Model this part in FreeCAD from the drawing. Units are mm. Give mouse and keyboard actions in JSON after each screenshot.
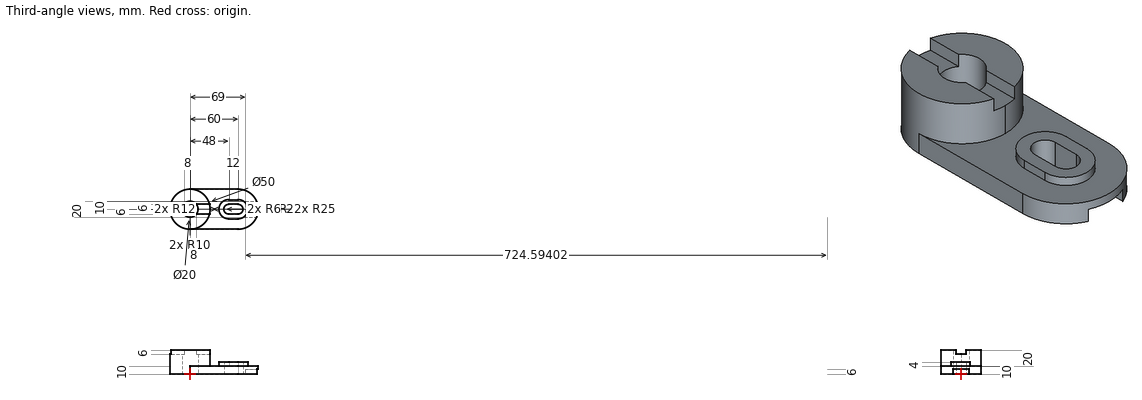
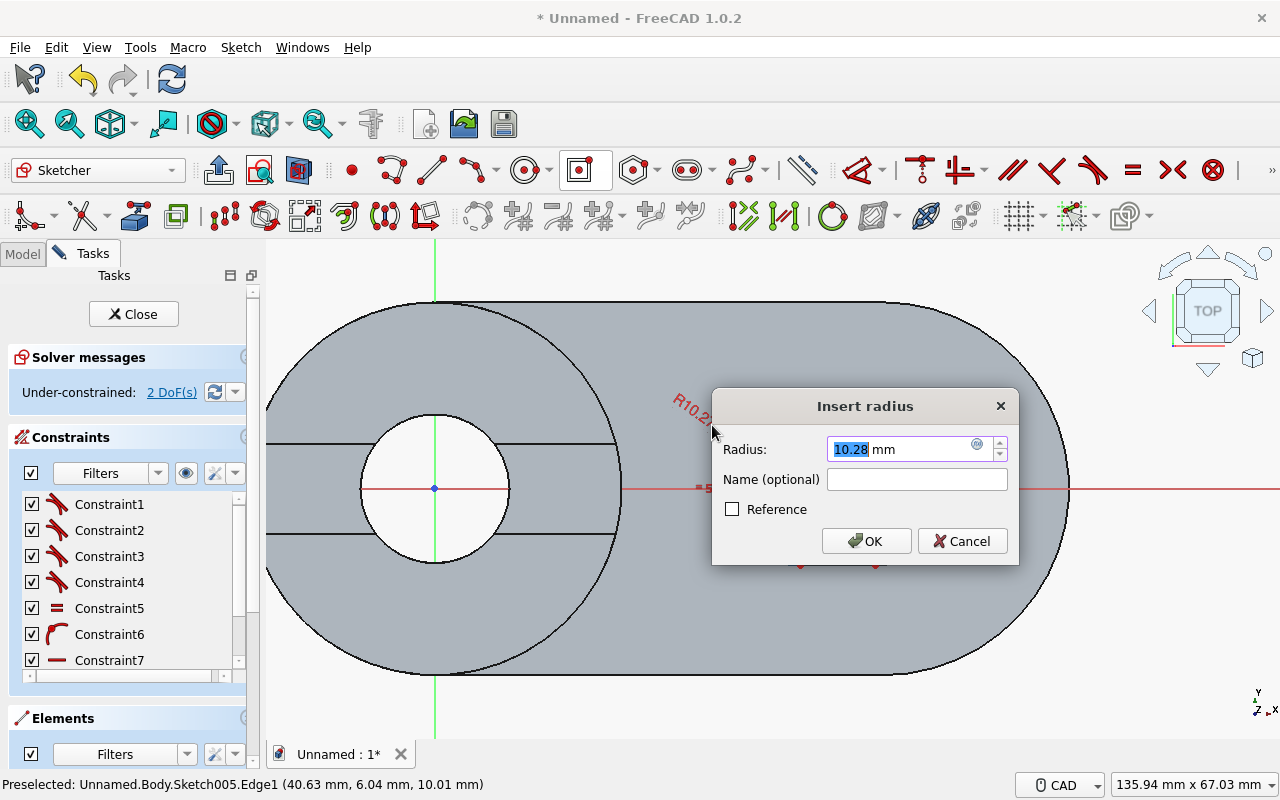
{"action": "type", "text": "12"}
{"action": "key", "text": "Return"}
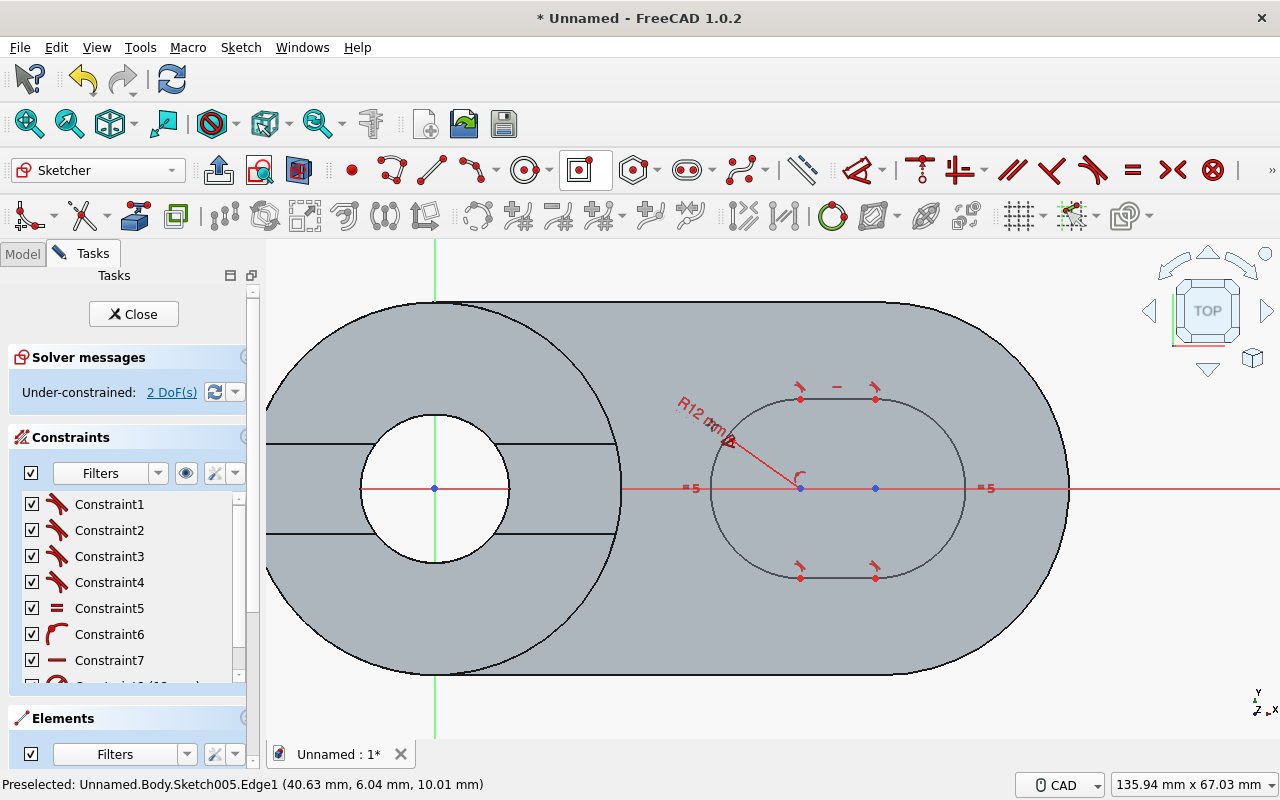
{"action": "left_click", "coordinate": [823, 399]}
{"action": "left_click", "coordinate": [838, 365]}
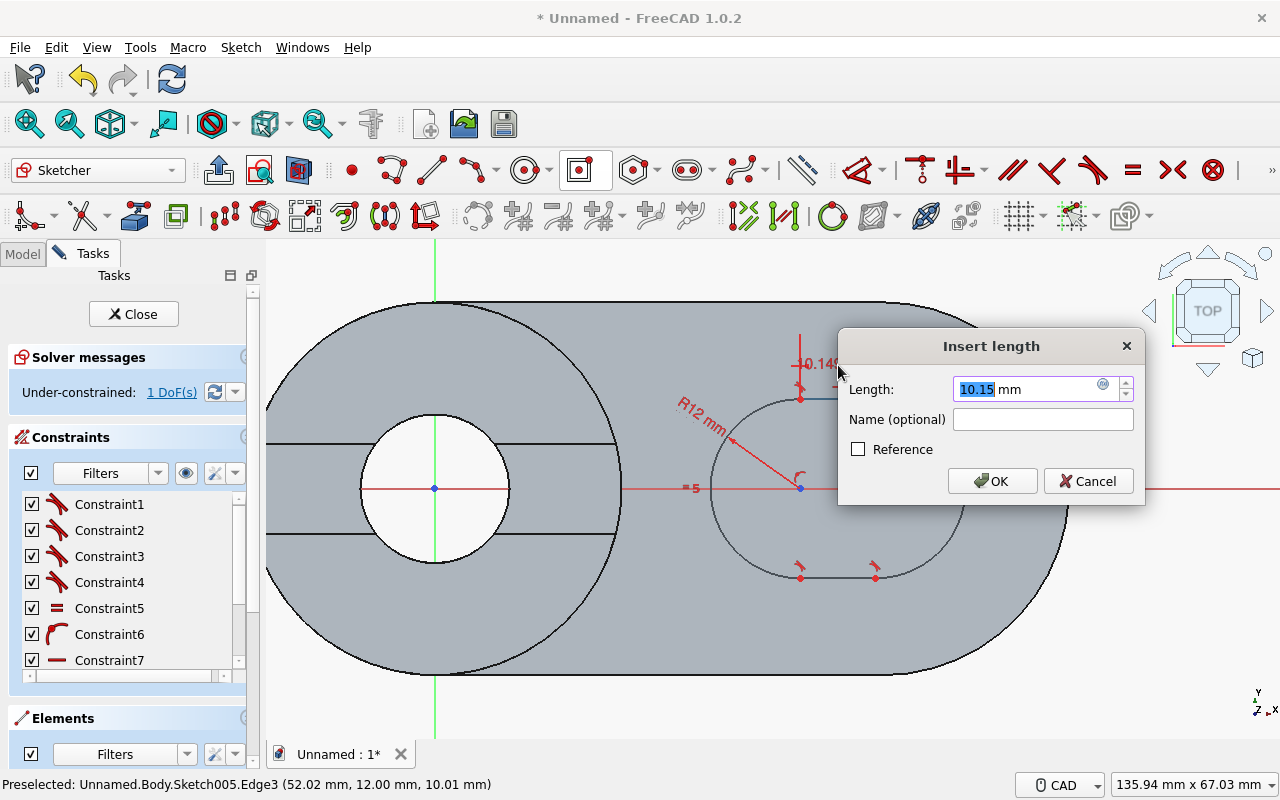
{"action": "type", "text": "12"}
{"action": "key", "text": "Return"}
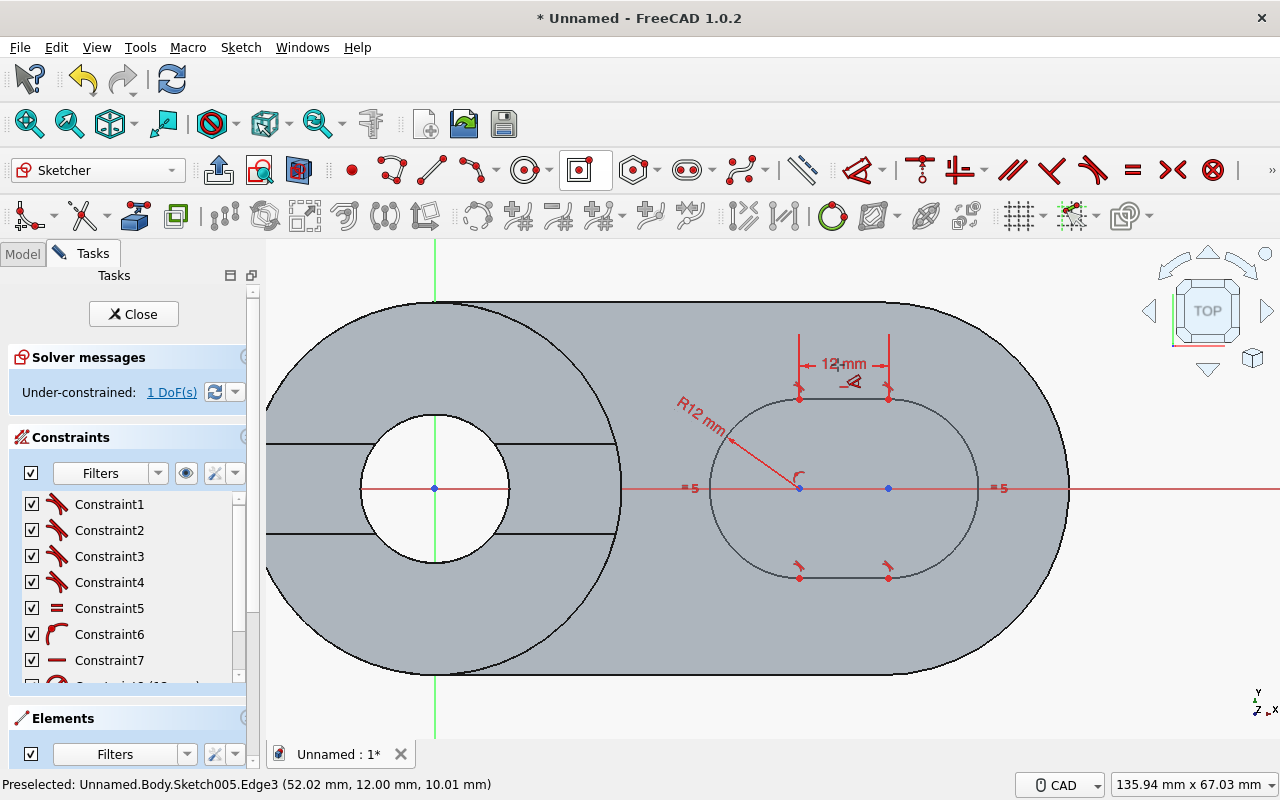
{"action": "left_click", "coordinate": [799, 399]}
{"action": "left_click", "coordinate": [617, 365]}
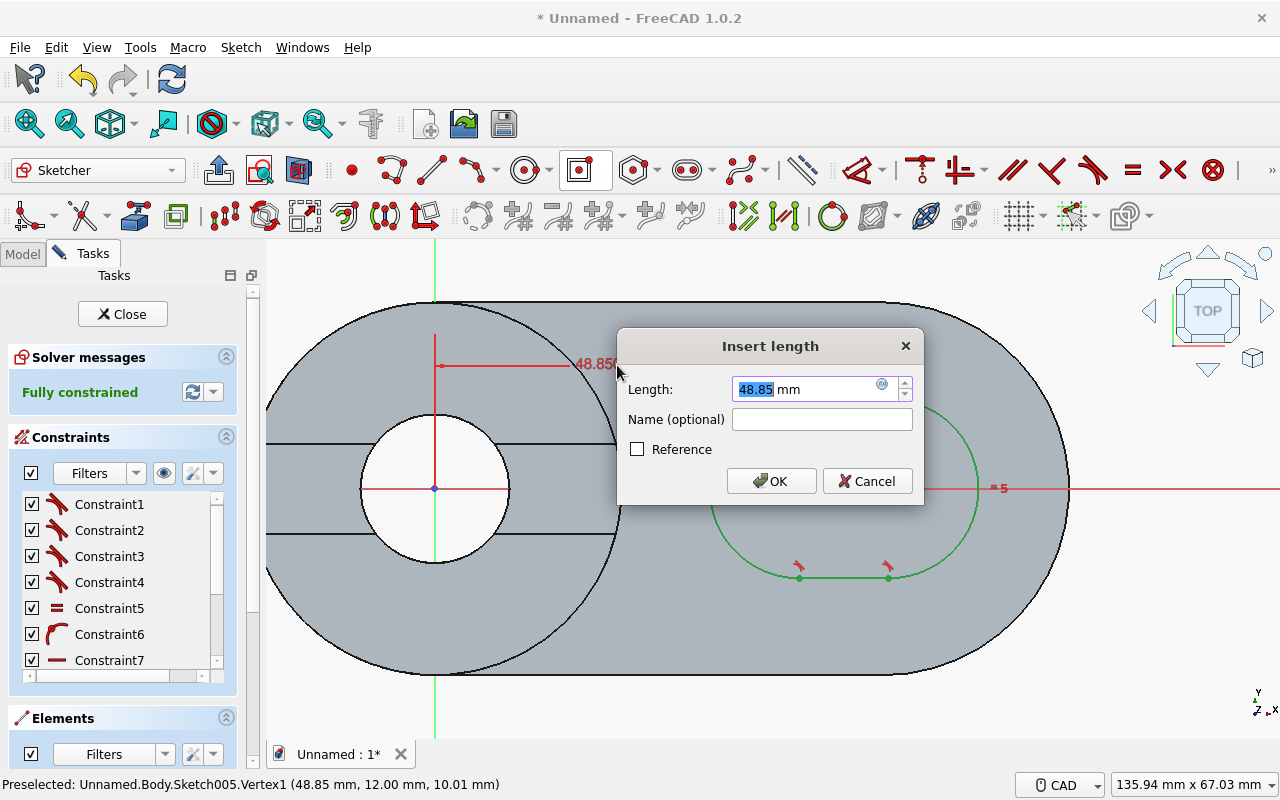
{"action": "type", "text": "48"}
{"action": "key", "text": "Return"}
{"action": "key", "text": "Escape"}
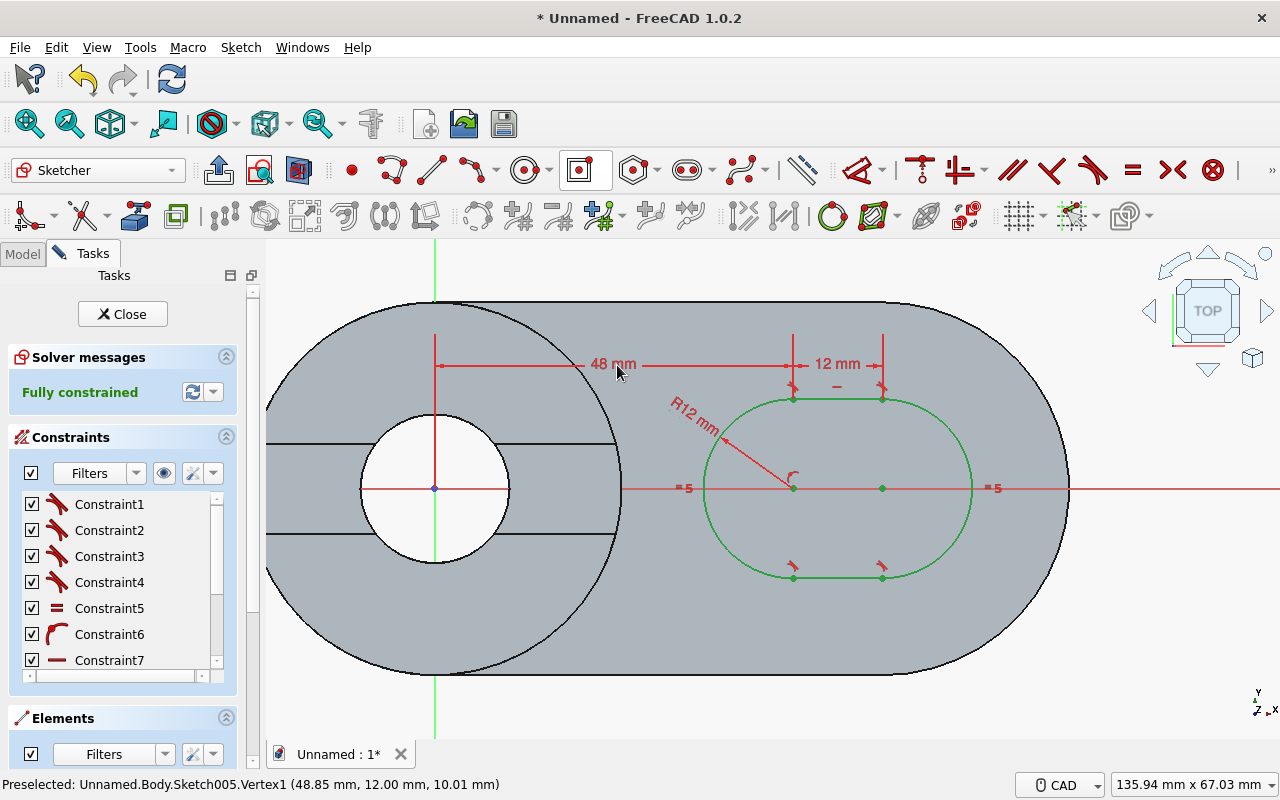
{"action": "left_click", "coordinate": [123, 314]}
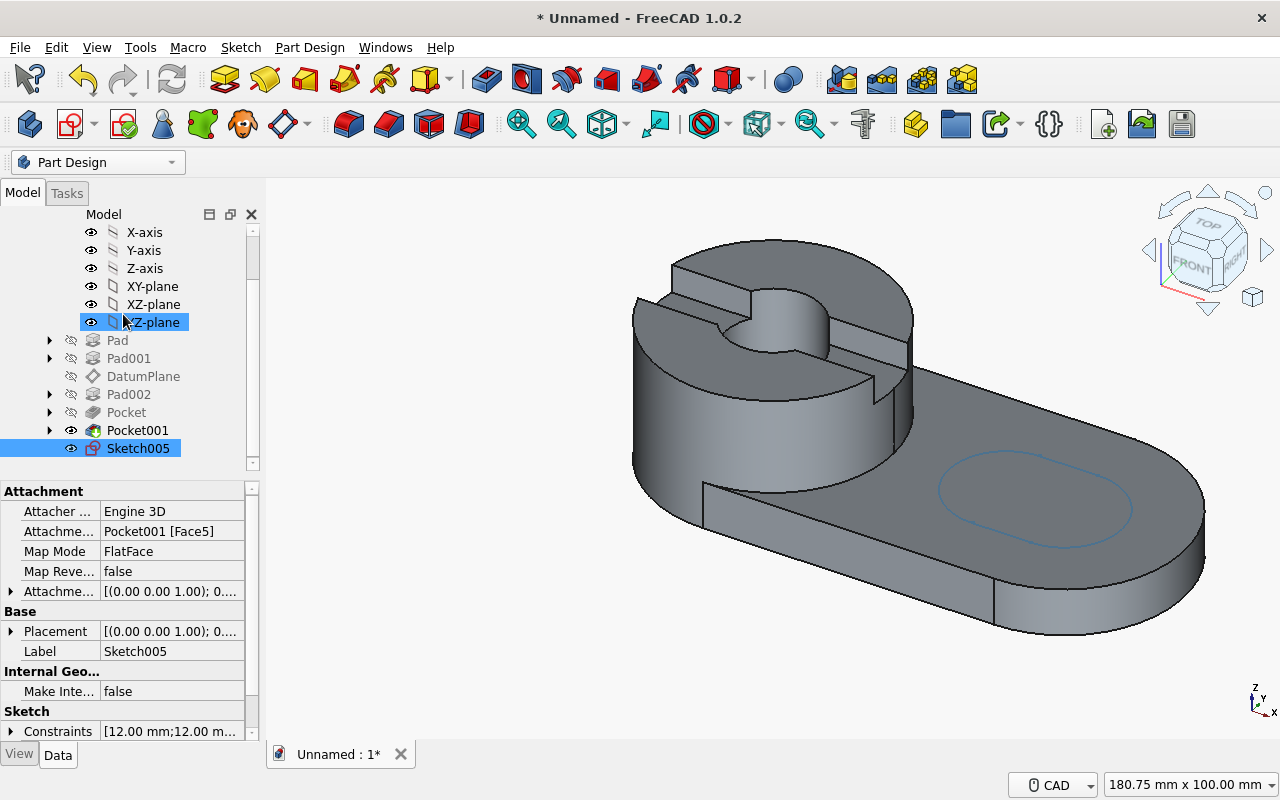
{"action": "left_click", "coordinate": [226, 80]}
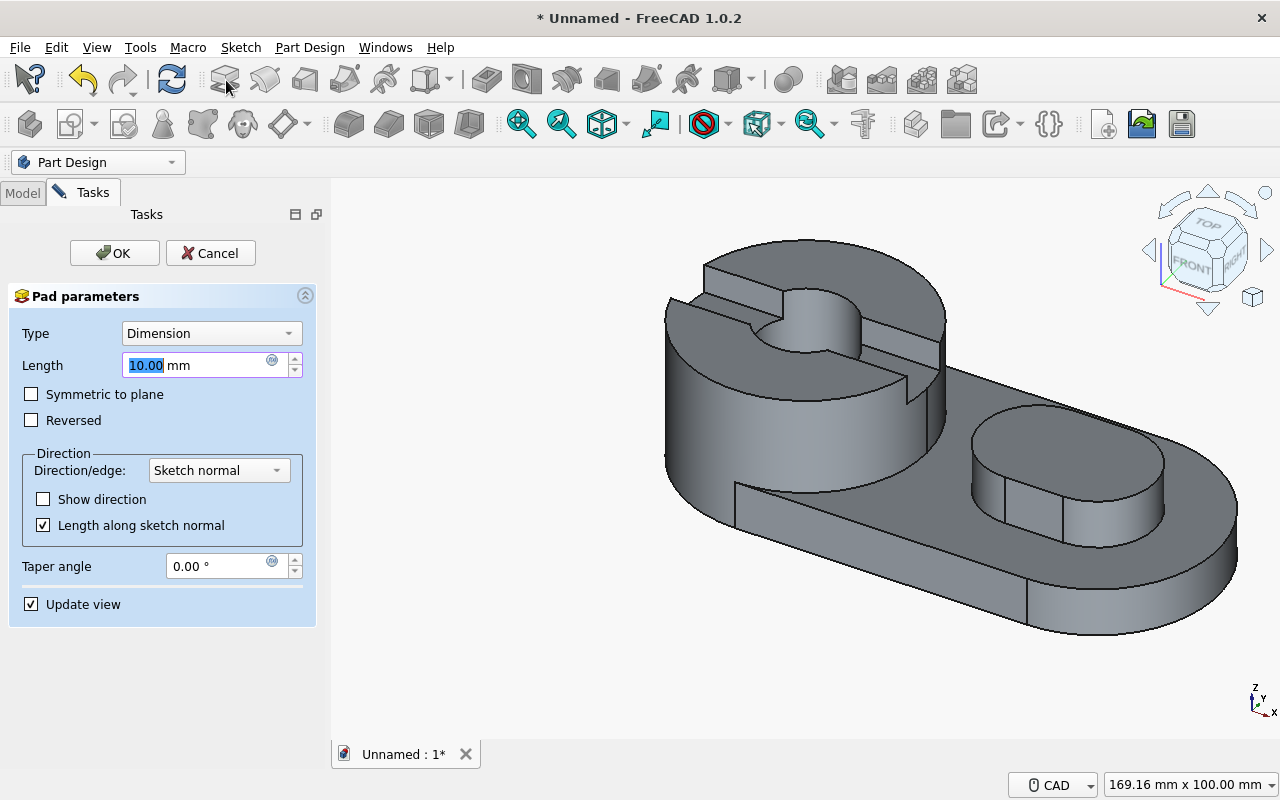
{"action": "type", "text": "4"}
{"action": "key", "text": "Tab"}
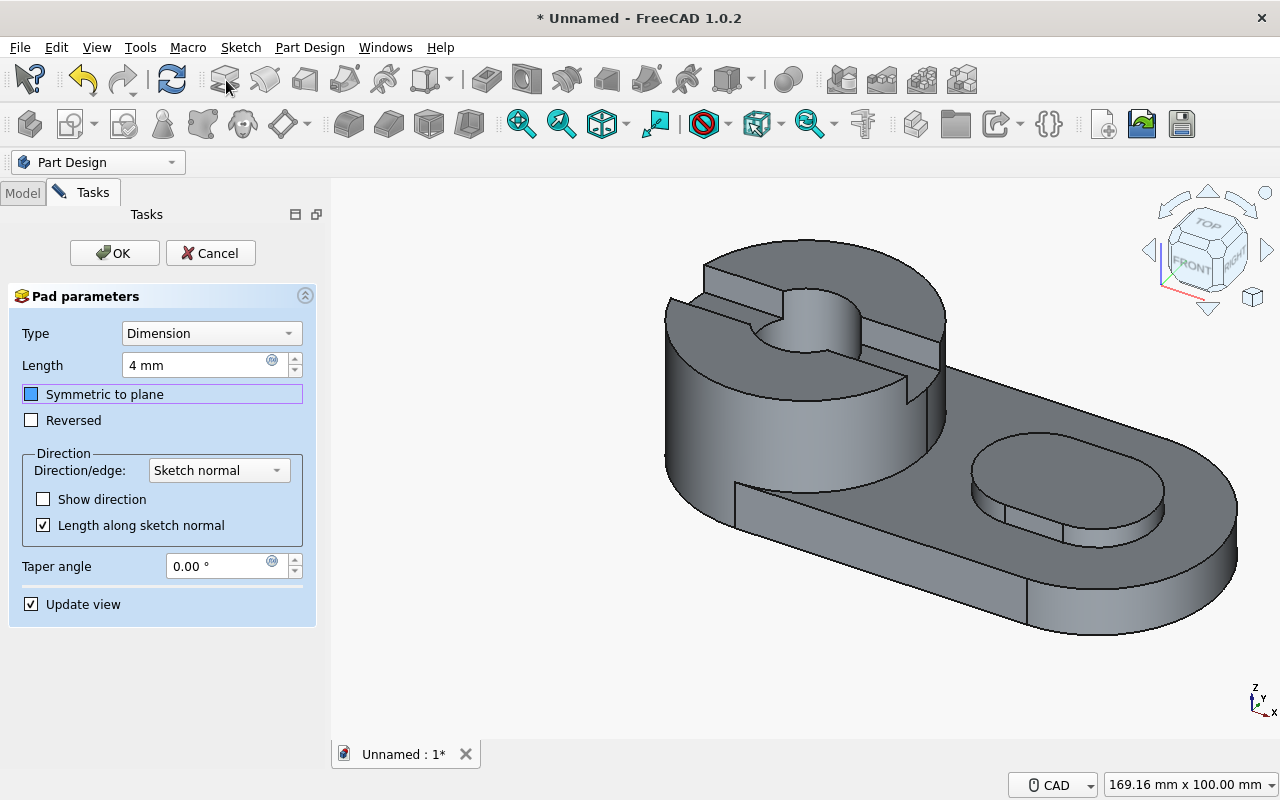
{"action": "left_click", "coordinate": [115, 253]}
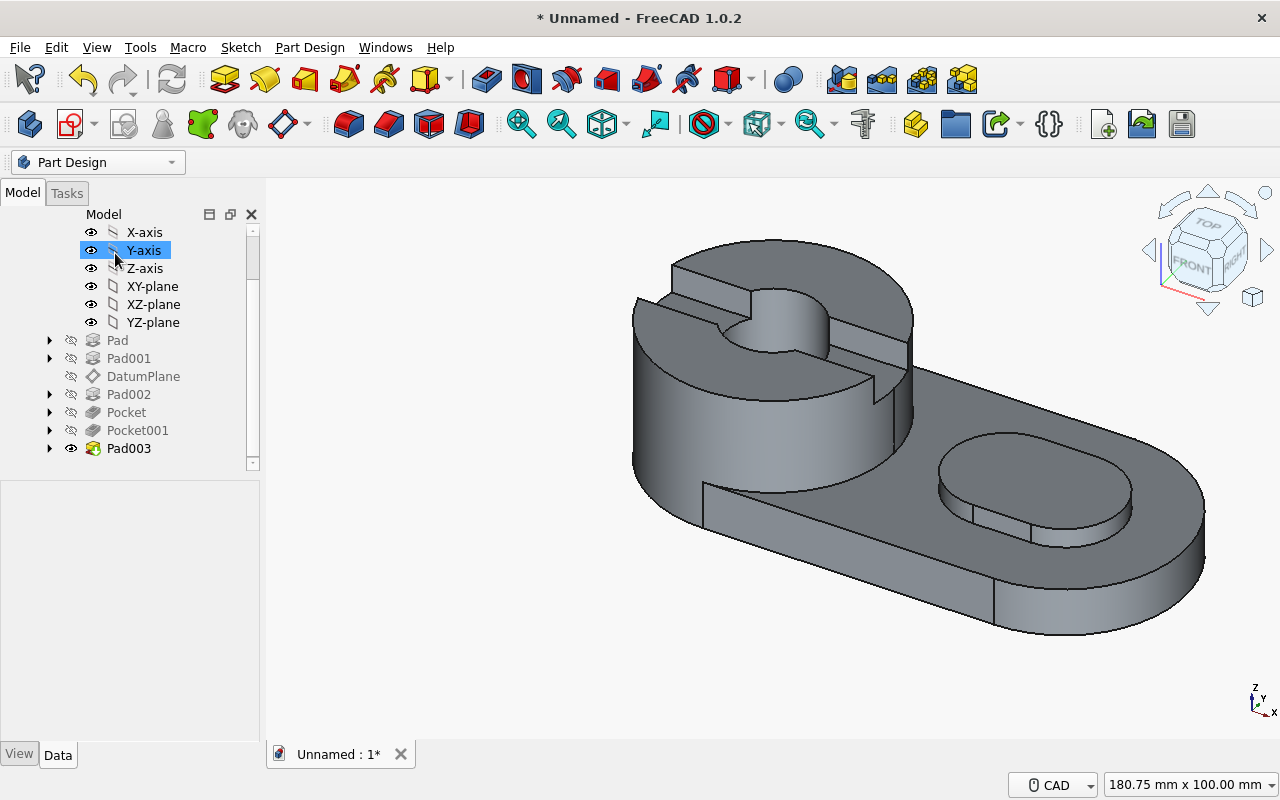
{"action": "left_click", "coordinate": [1010, 472]}